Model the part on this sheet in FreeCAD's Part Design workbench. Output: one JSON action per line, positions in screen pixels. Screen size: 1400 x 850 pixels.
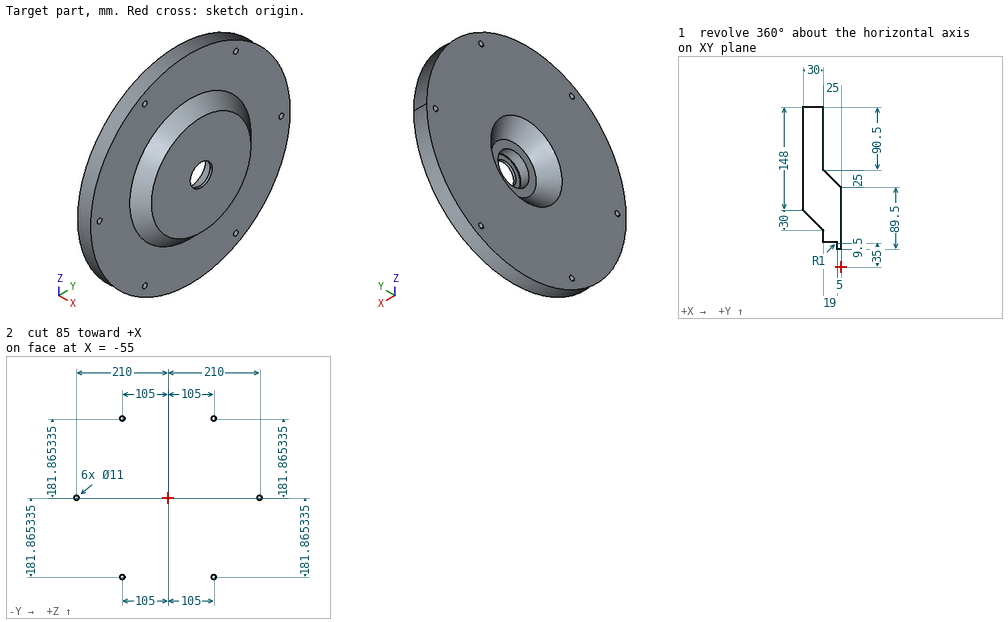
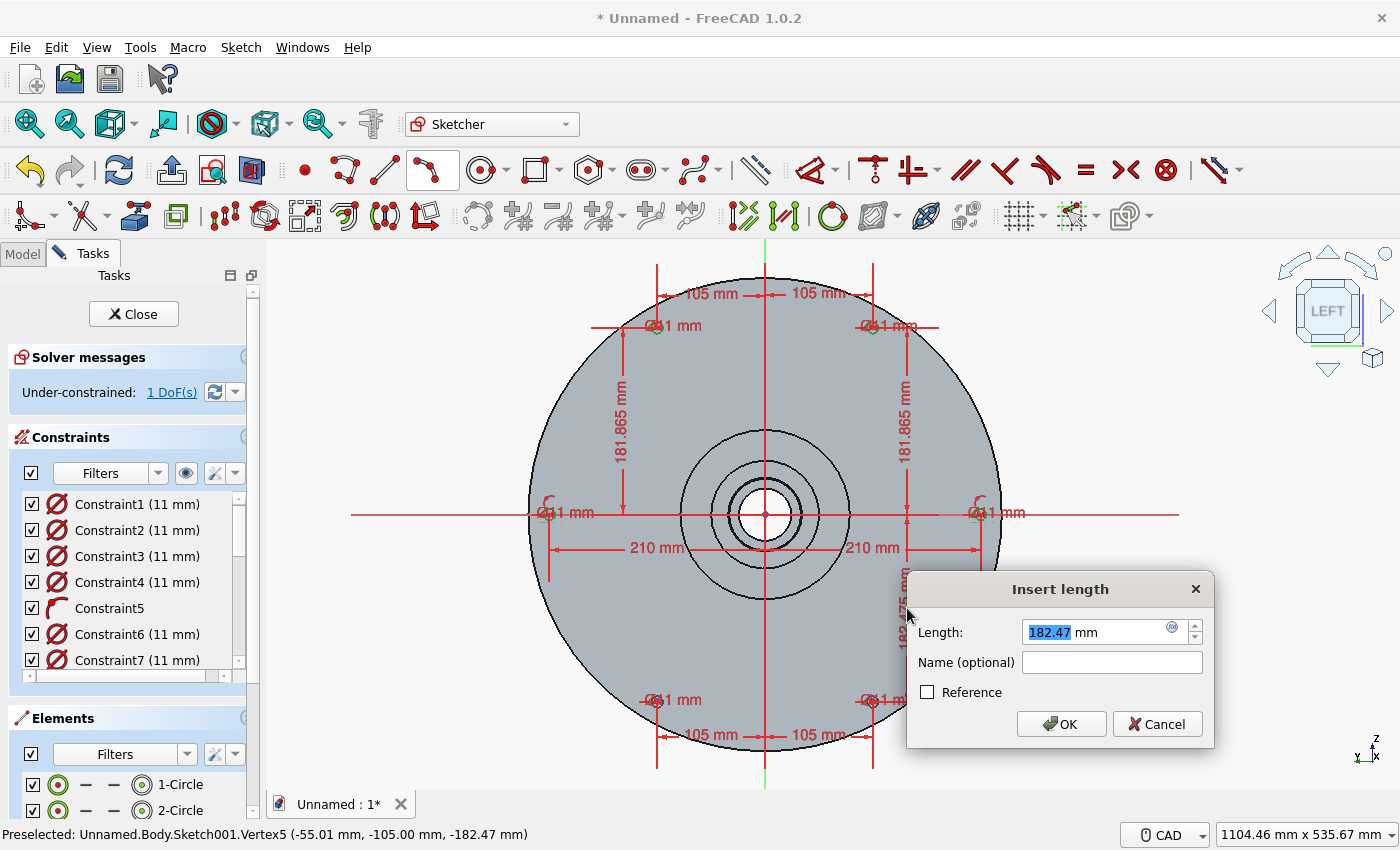
{"action": "type", "text": "181.865335"}
{"action": "key", "text": "Return"}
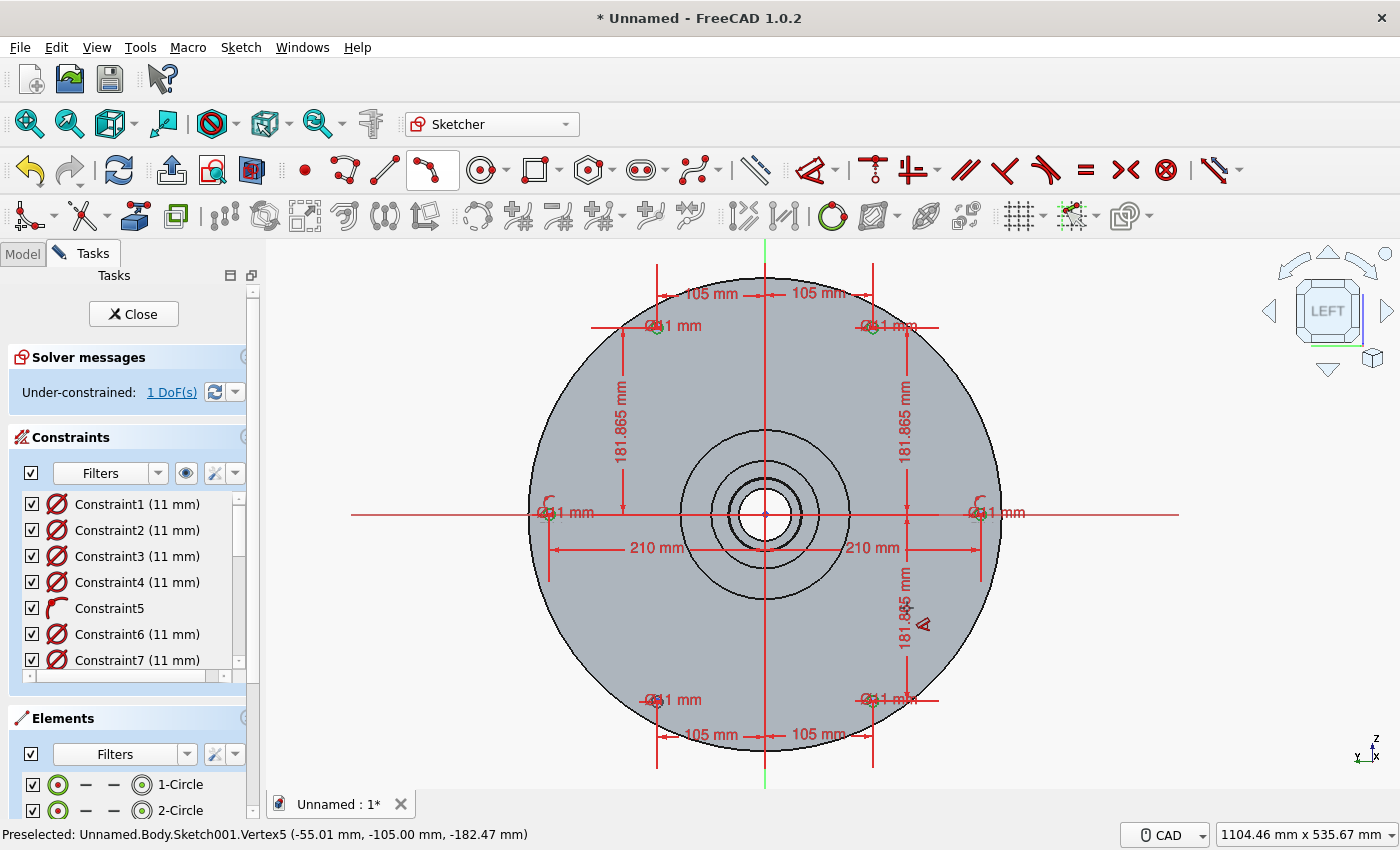
{"action": "left_click", "coordinate": [657, 702]}
{"action": "left_click", "coordinate": [623, 608]}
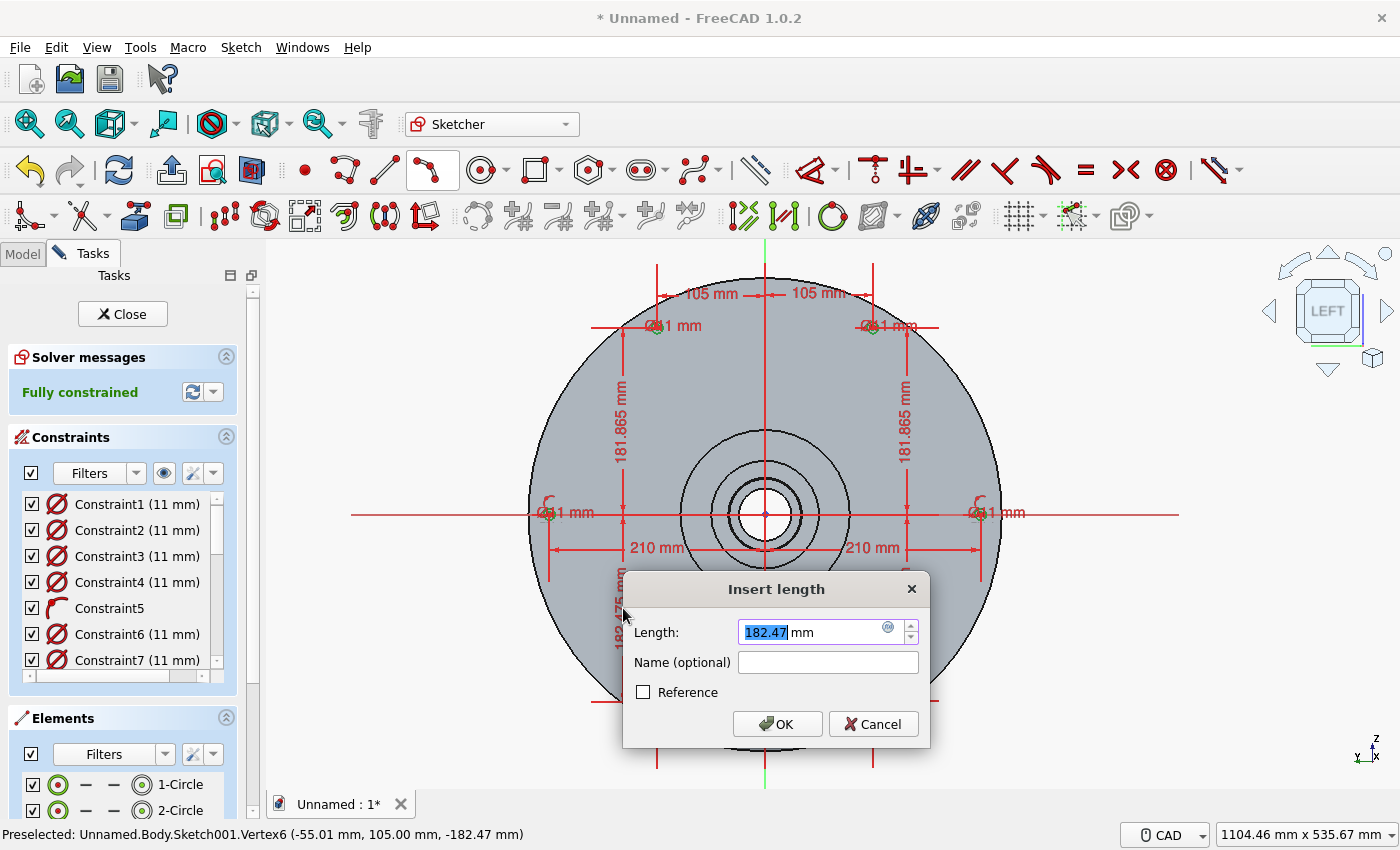
{"action": "type", "text": "181.865335"}
{"action": "key", "text": "Return"}
{"action": "key", "text": "Escape"}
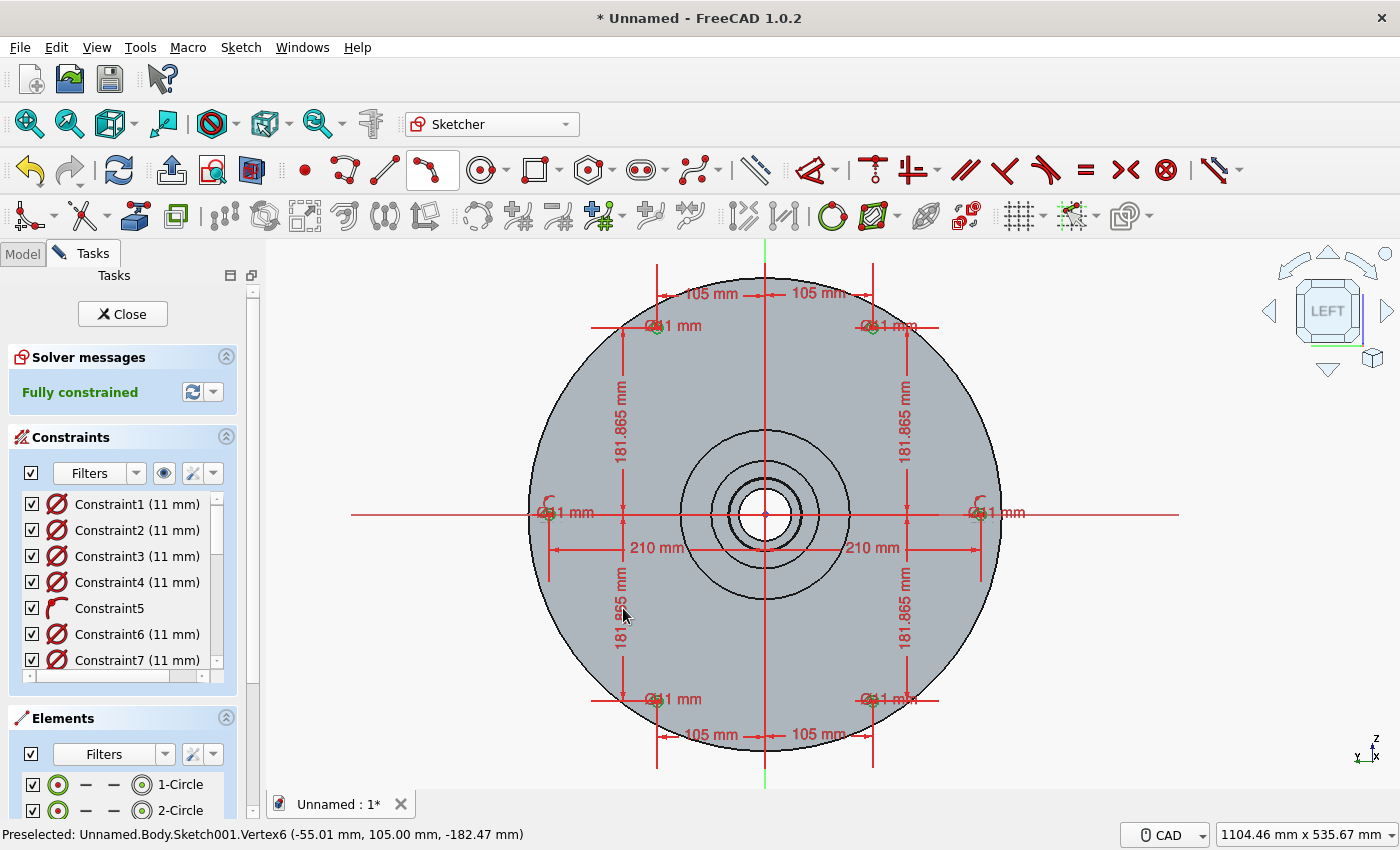
{"action": "left_click", "coordinate": [123, 314]}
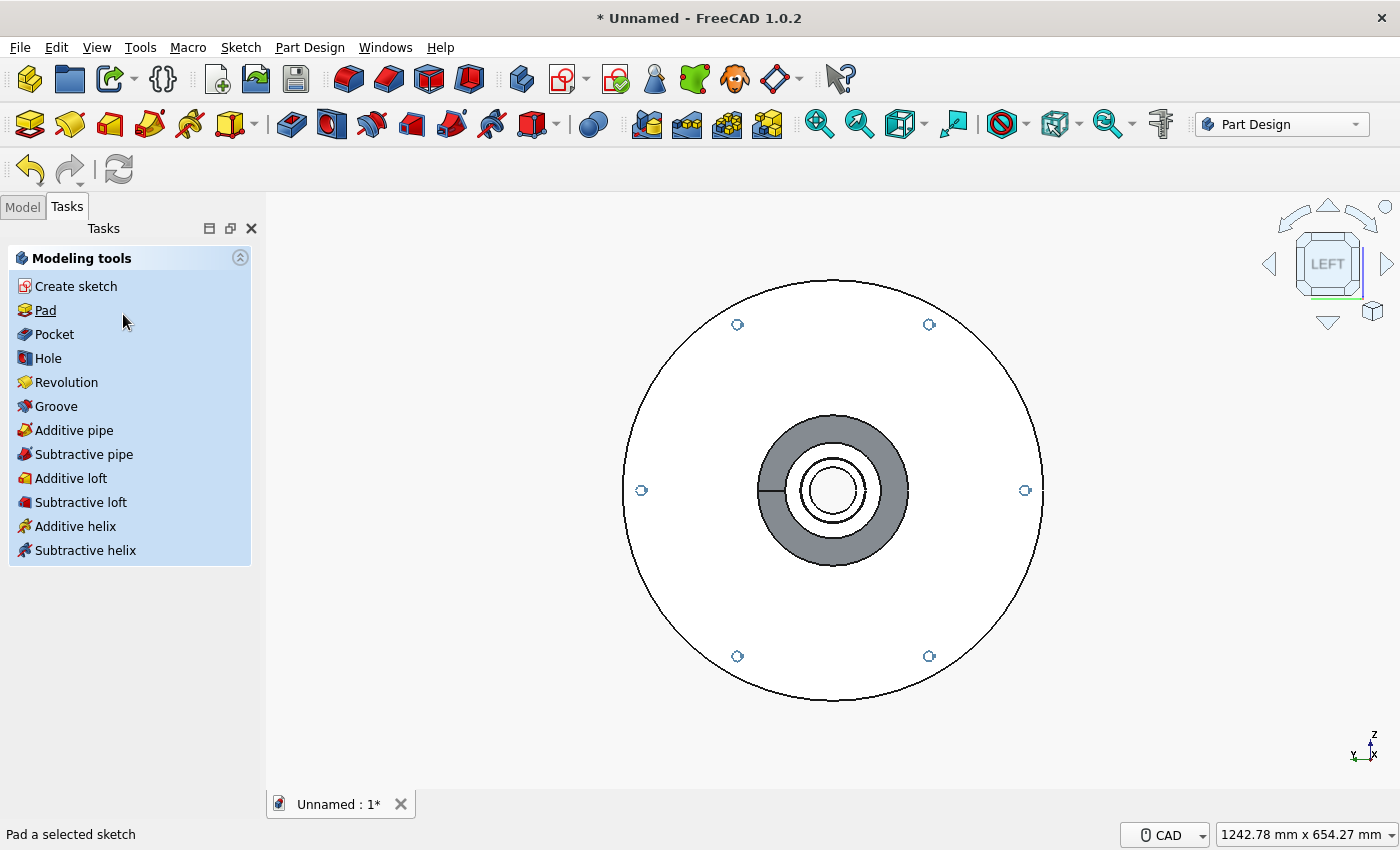
{"action": "left_click", "coordinate": [292, 124]}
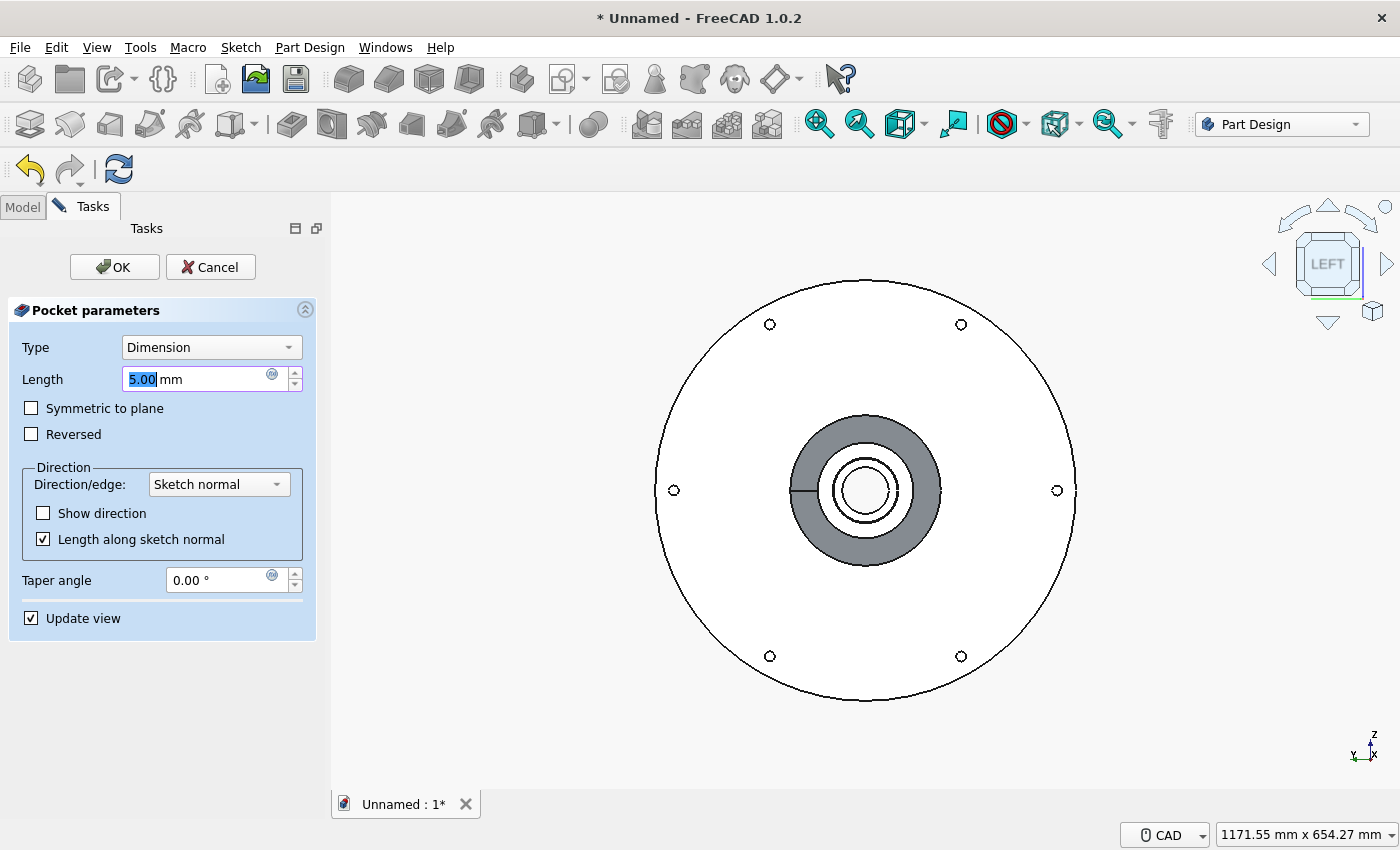
{"action": "type", "text": "85"}
{"action": "key", "text": "Tab"}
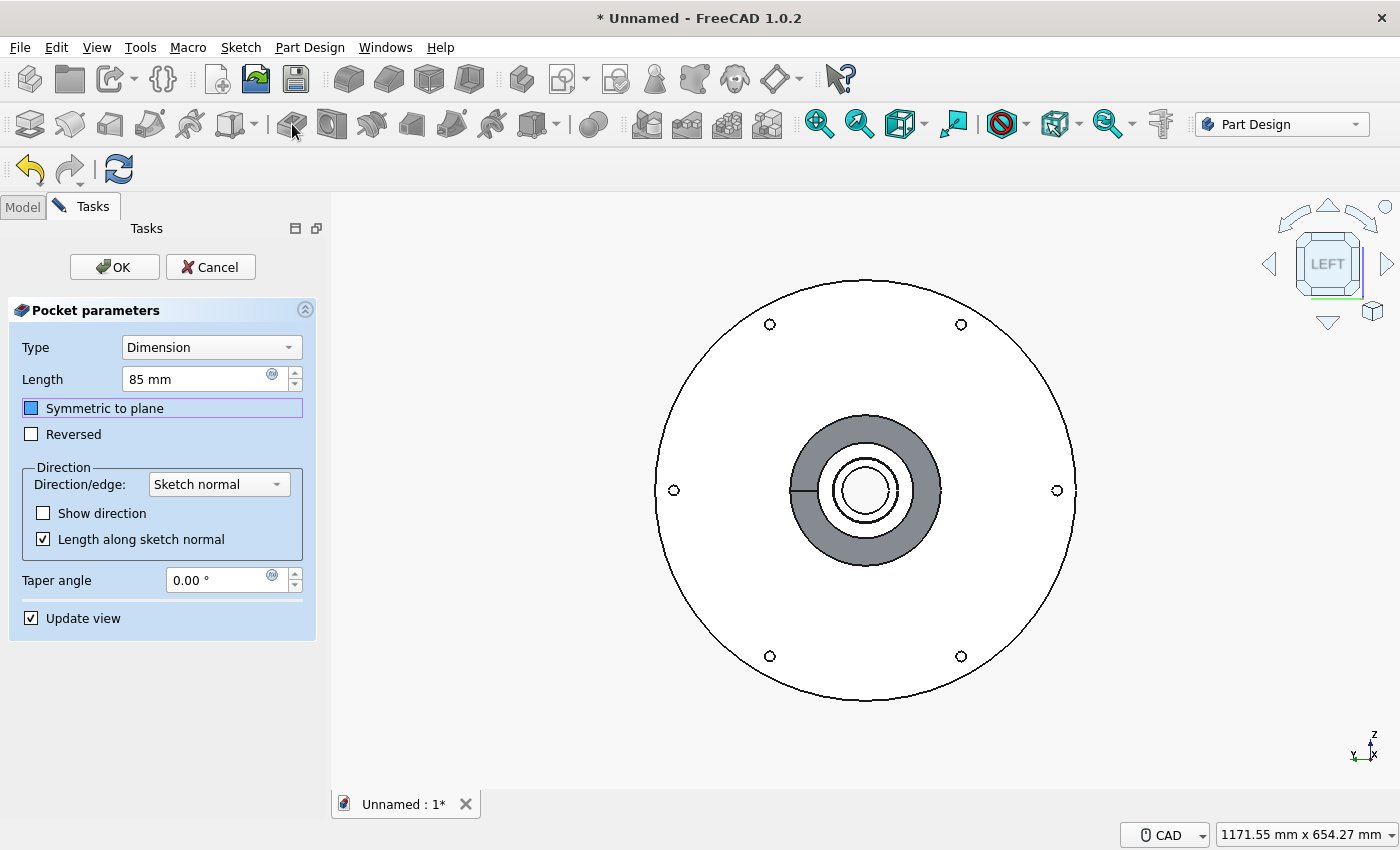
{"action": "left_click", "coordinate": [115, 267]}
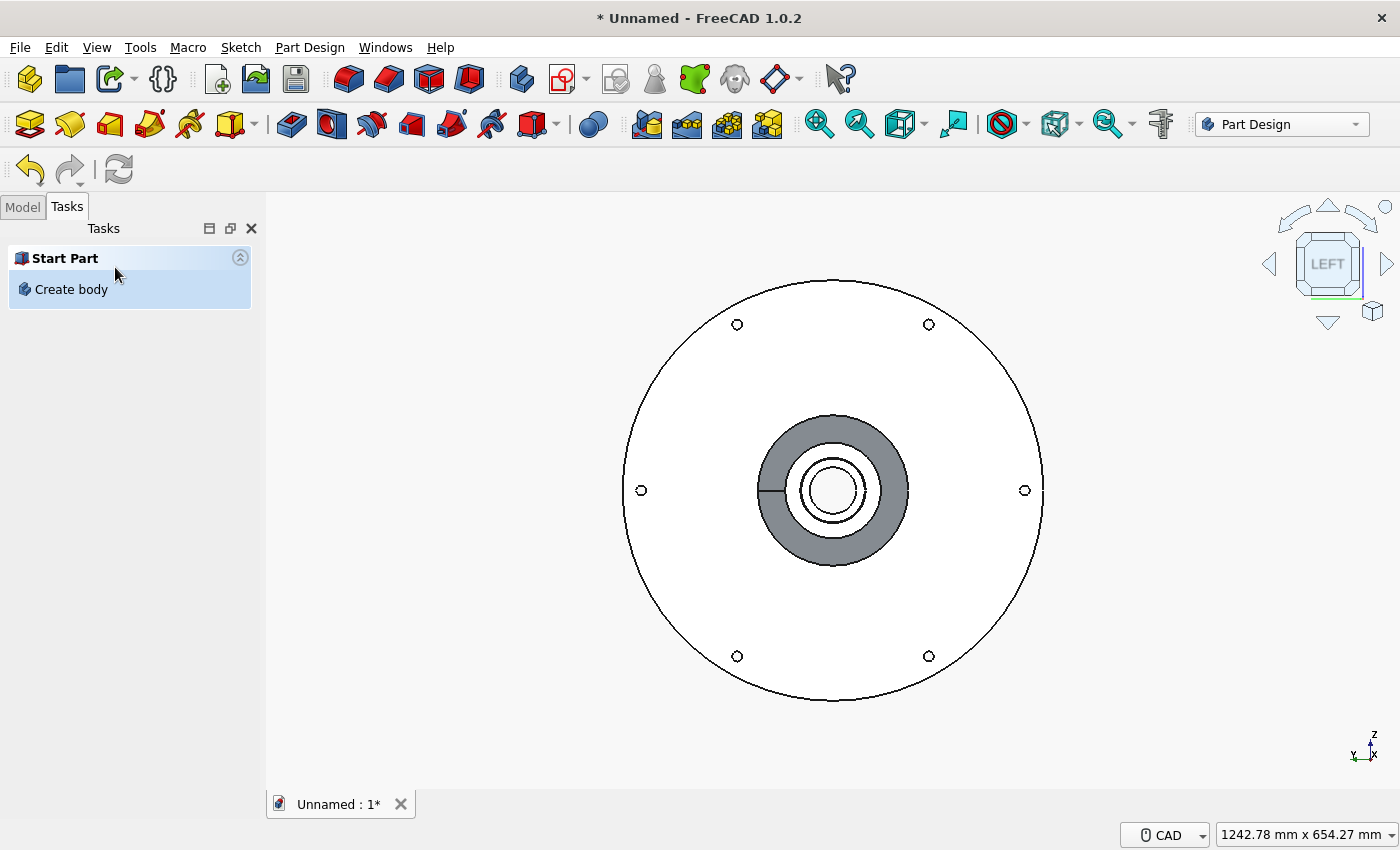
{"action": "key", "text": "0"}